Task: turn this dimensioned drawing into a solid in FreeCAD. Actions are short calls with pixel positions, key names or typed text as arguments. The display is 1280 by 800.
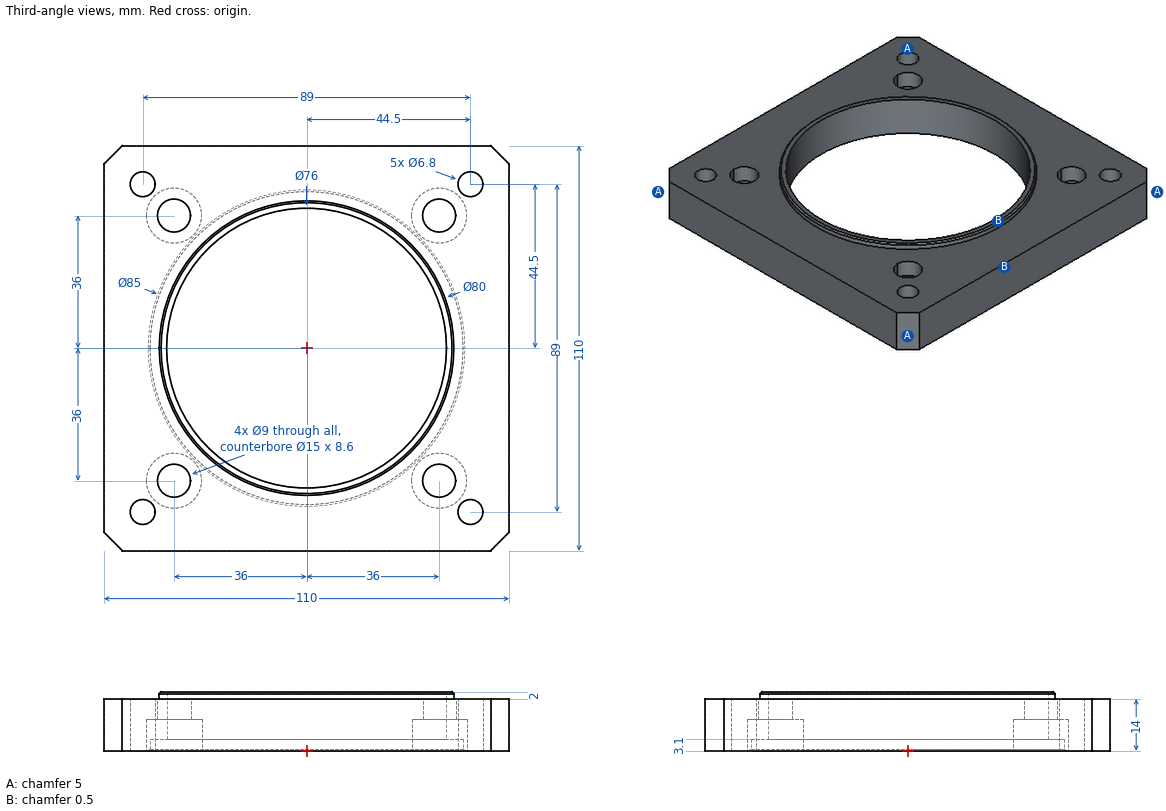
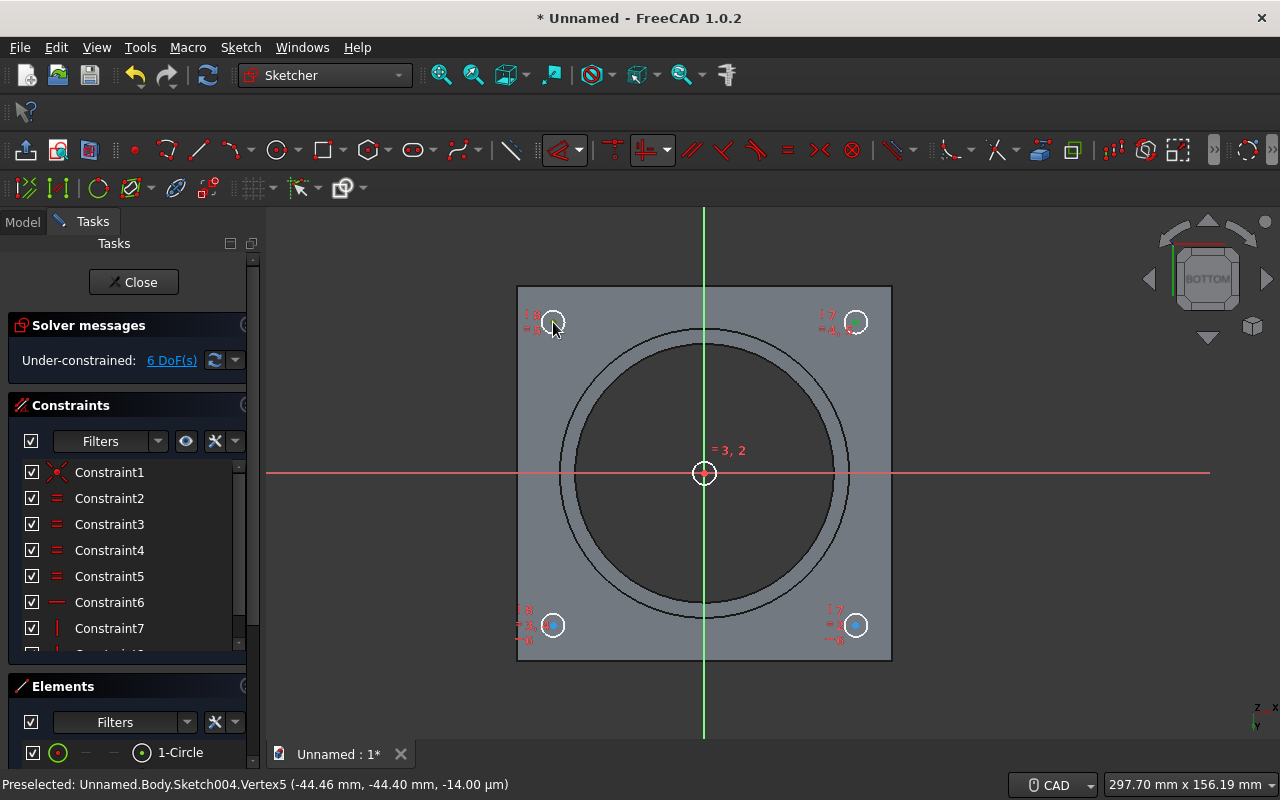
key(h)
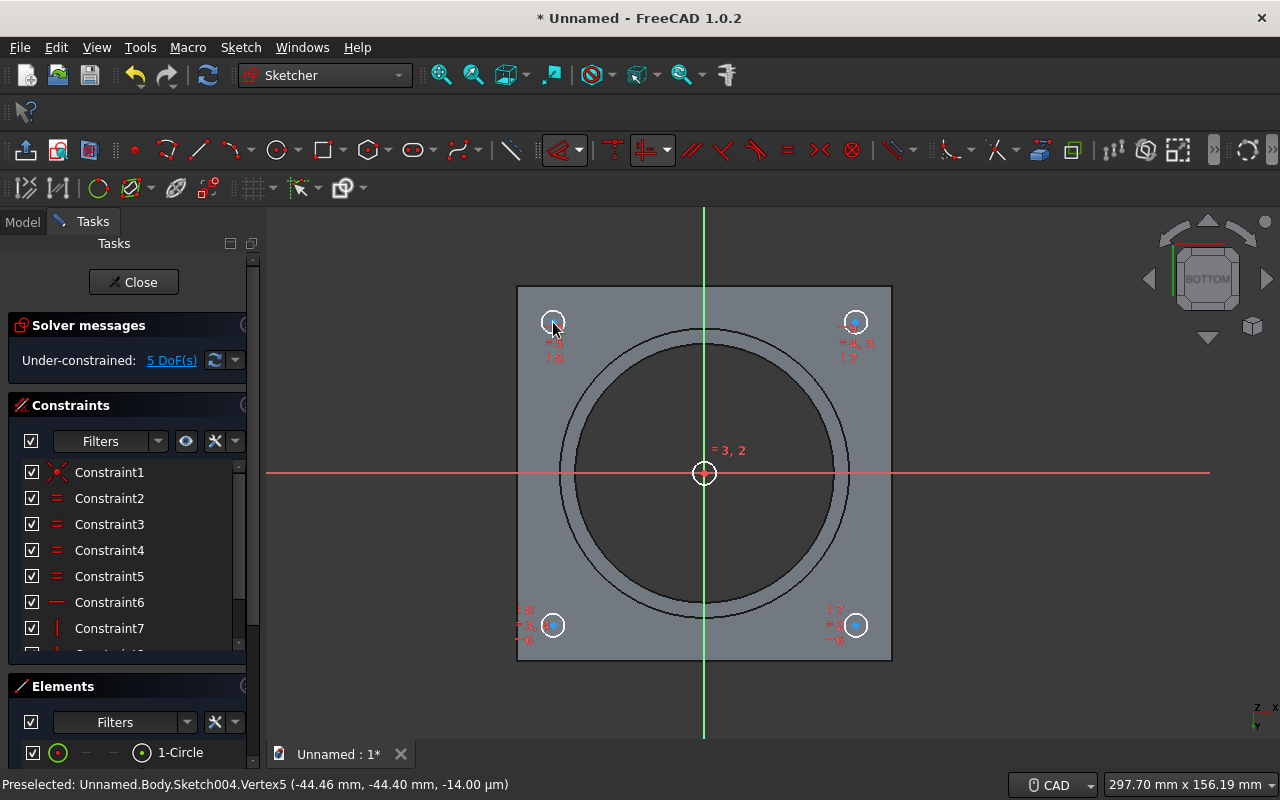
scroll(864, 617, up, 3)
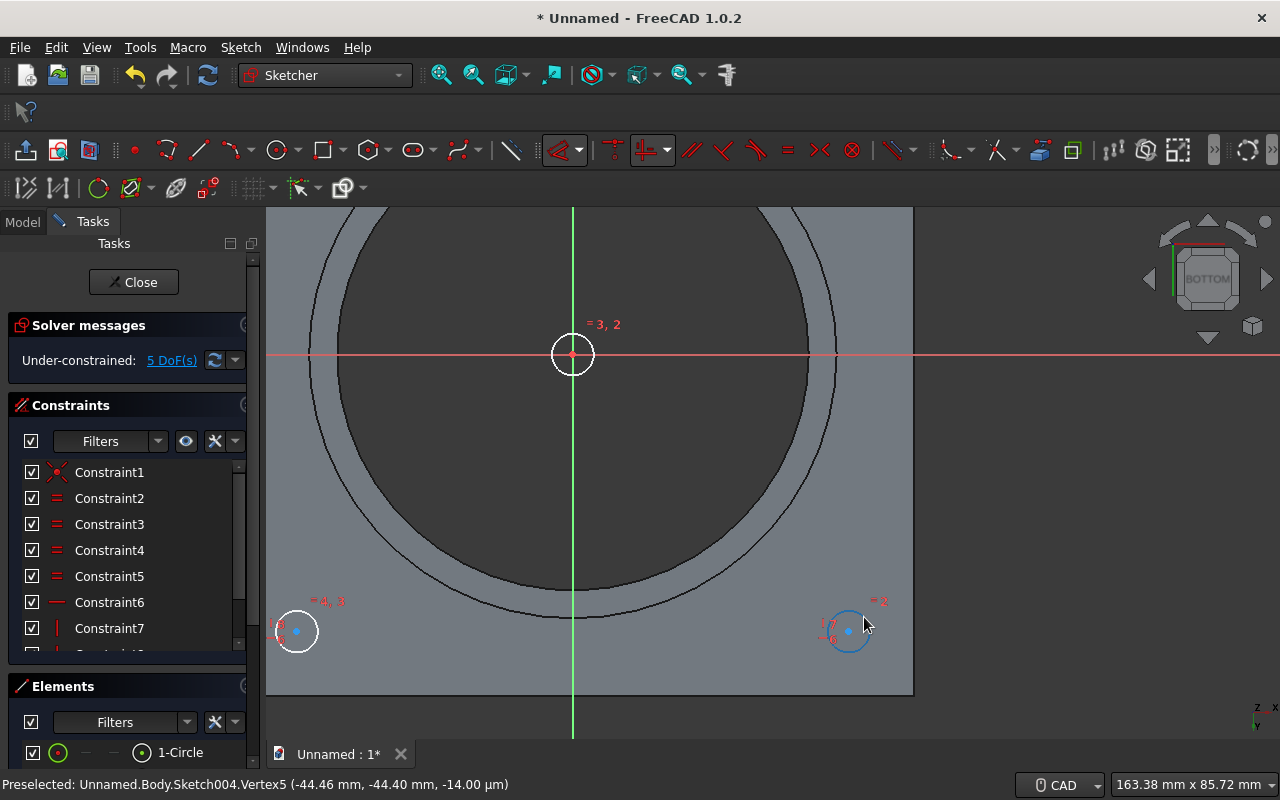
click(864, 617)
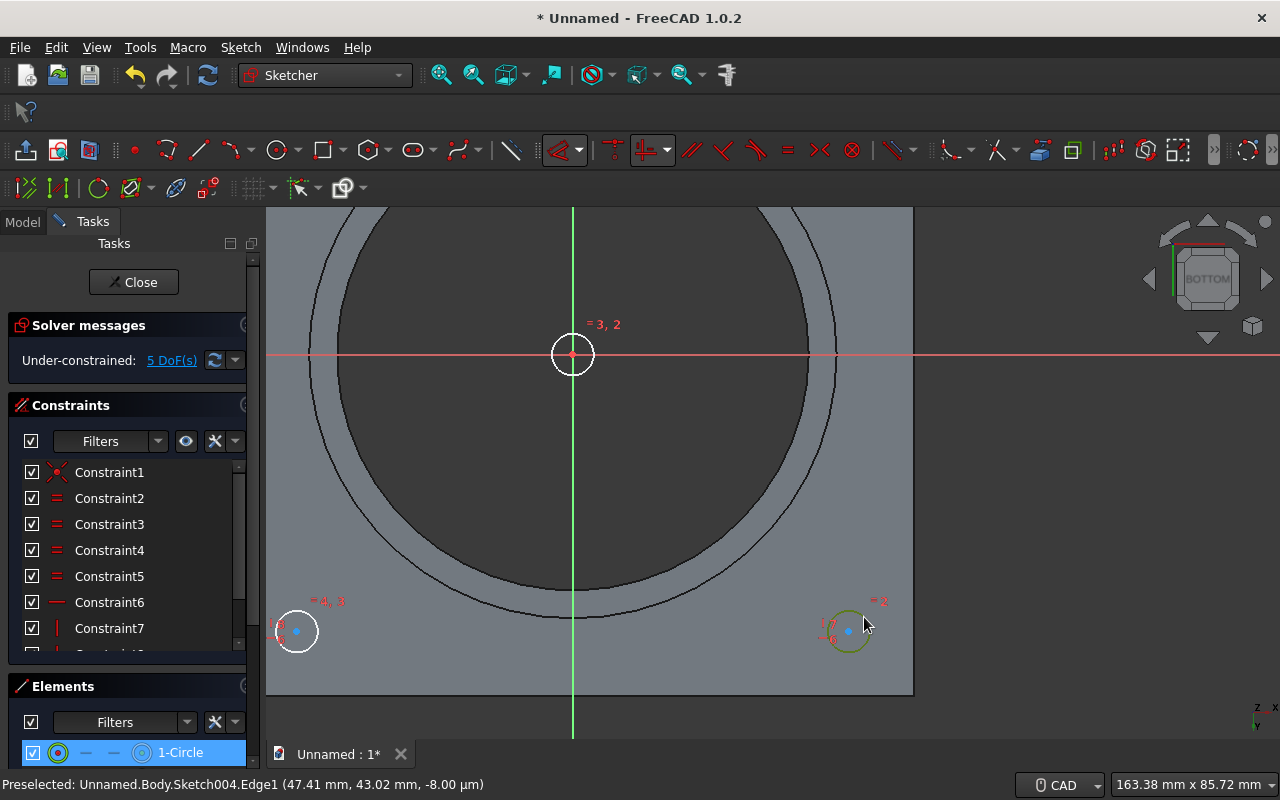
key(k)
key(o)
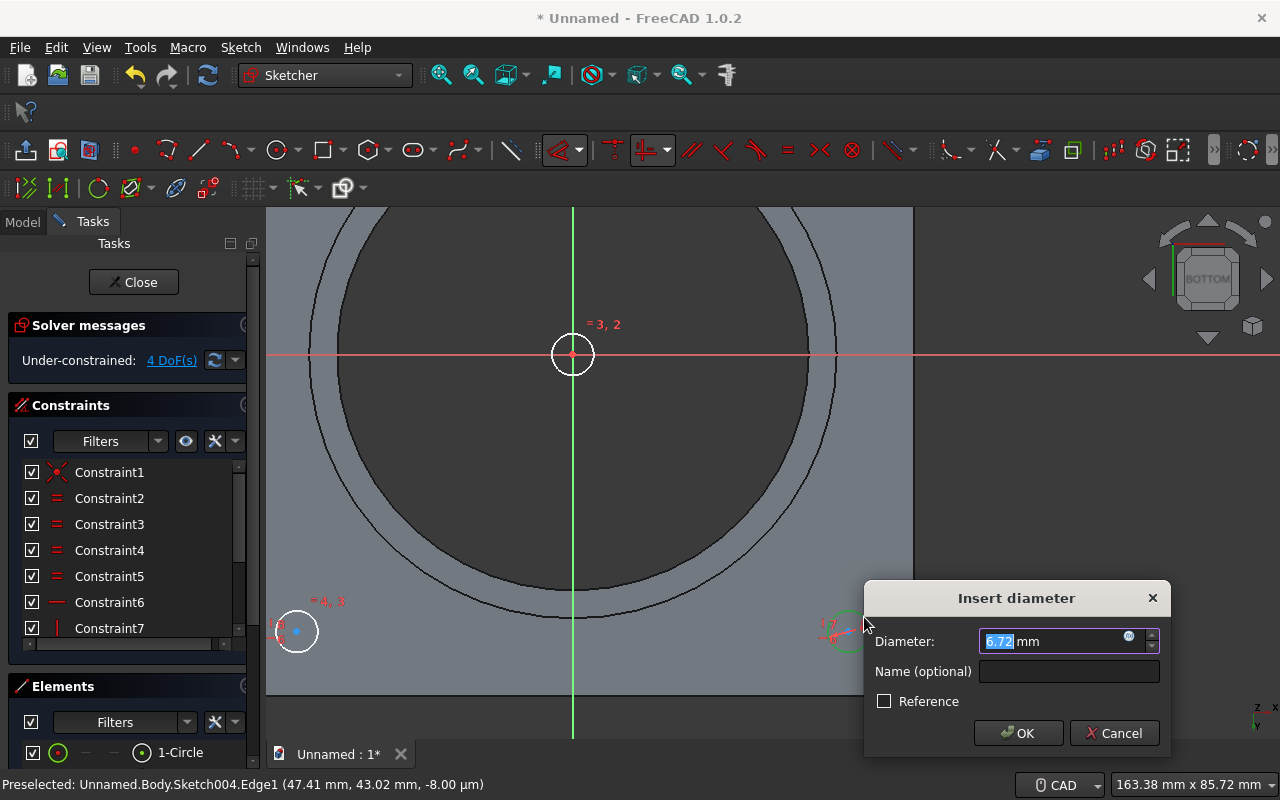
text(6.8)
key(Return)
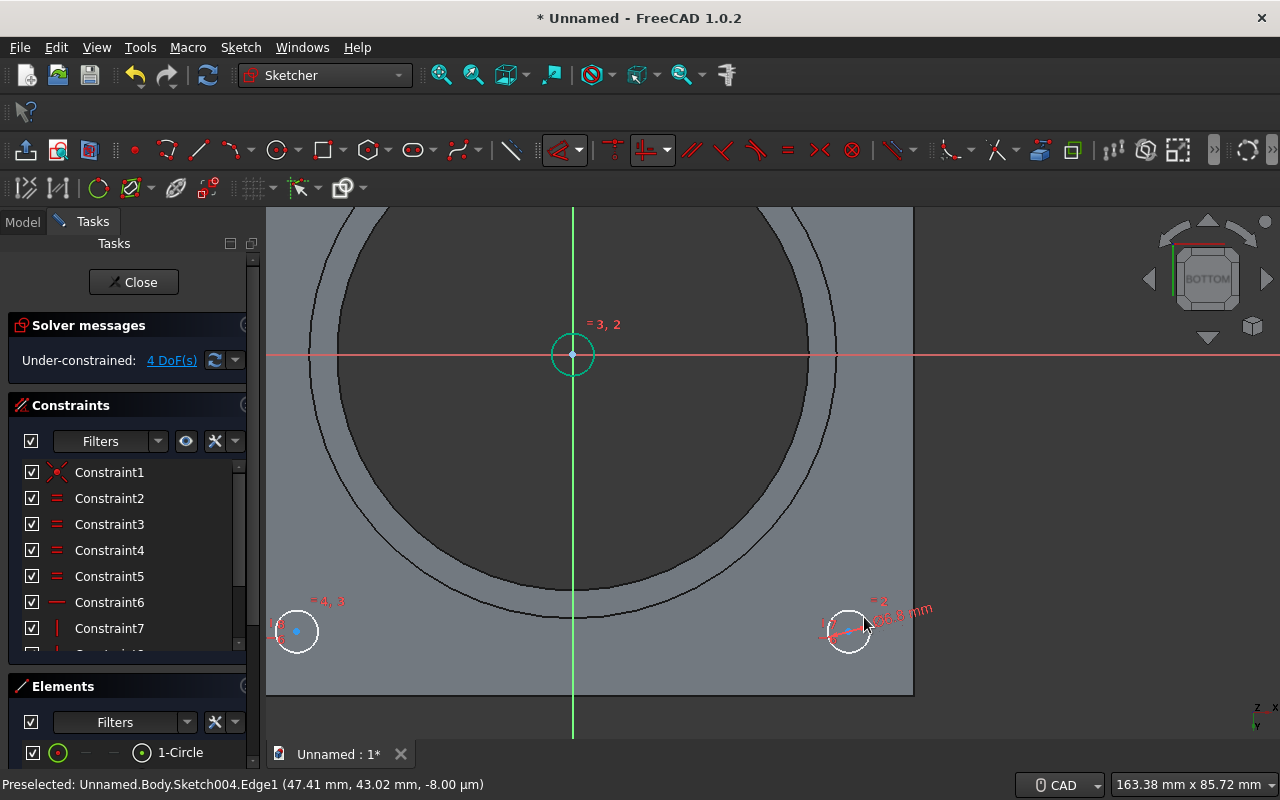
click(849, 632)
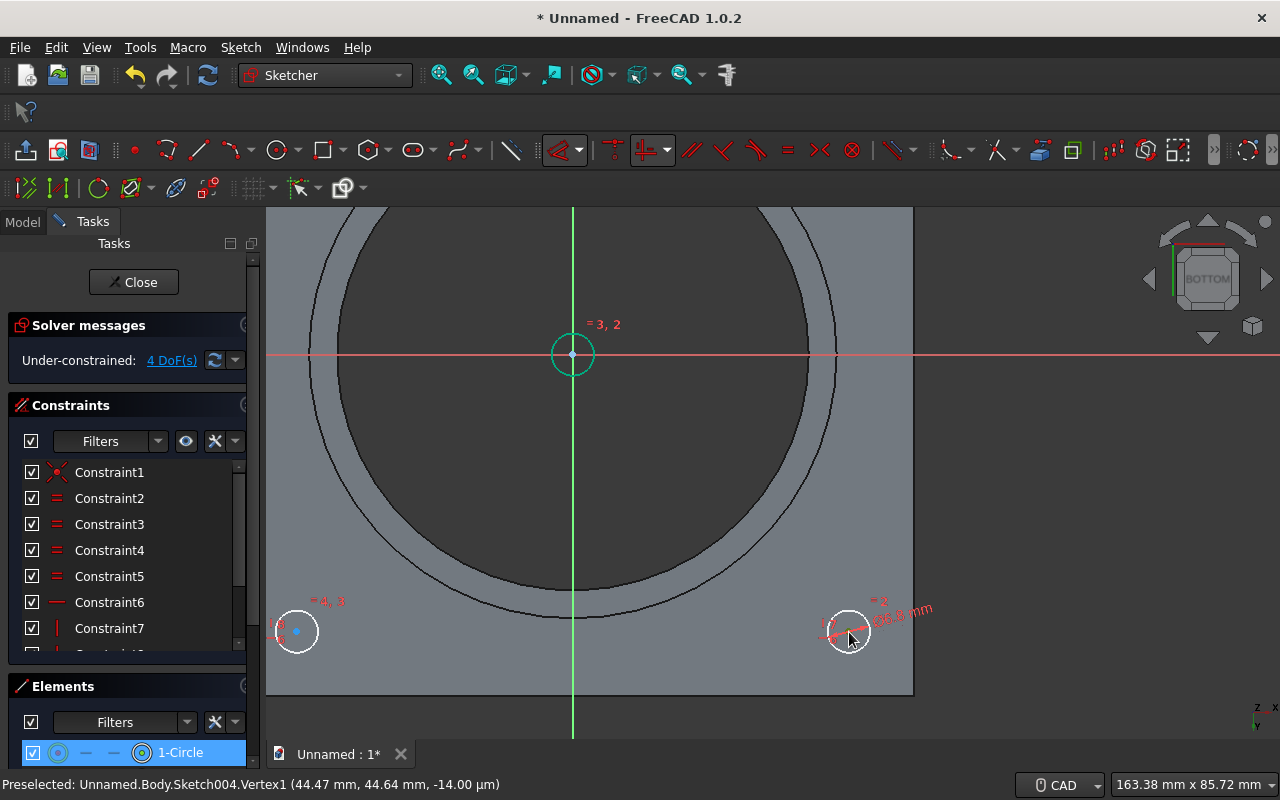
click(297, 632)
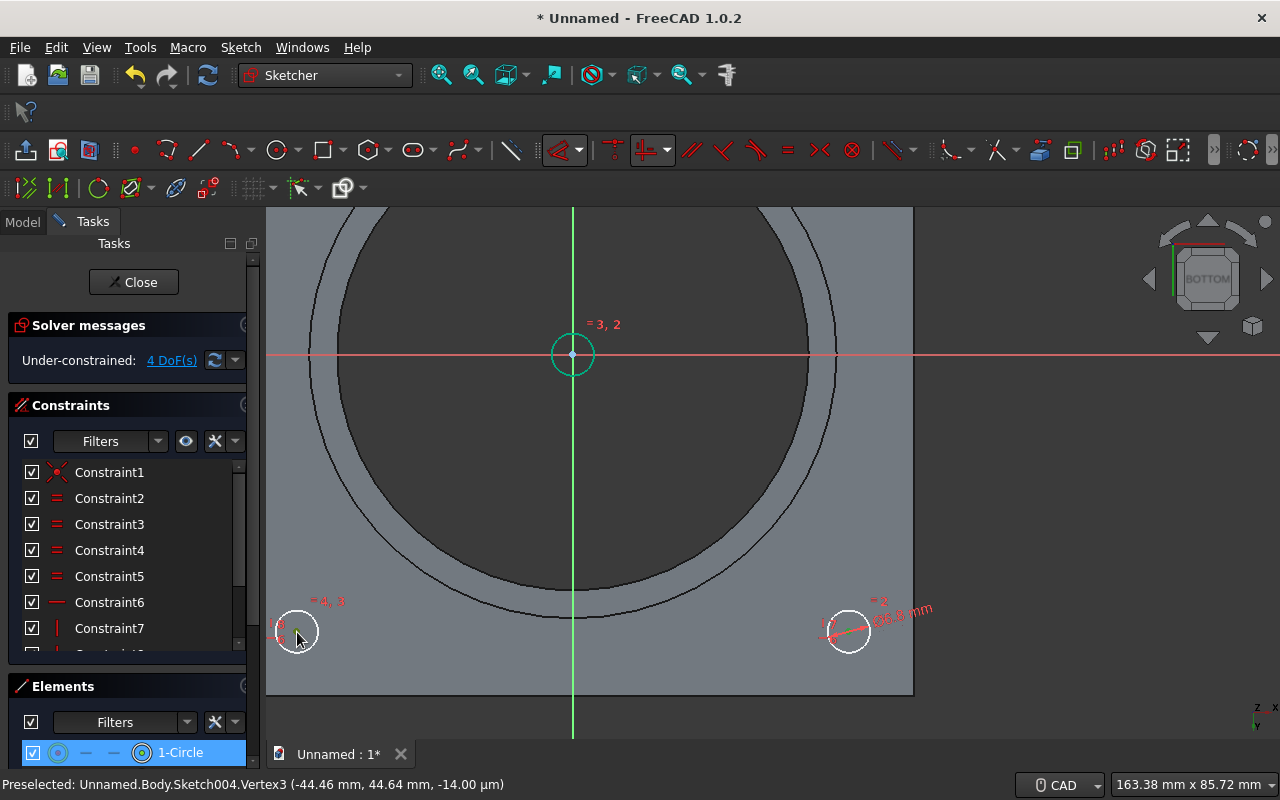
click(582, 150)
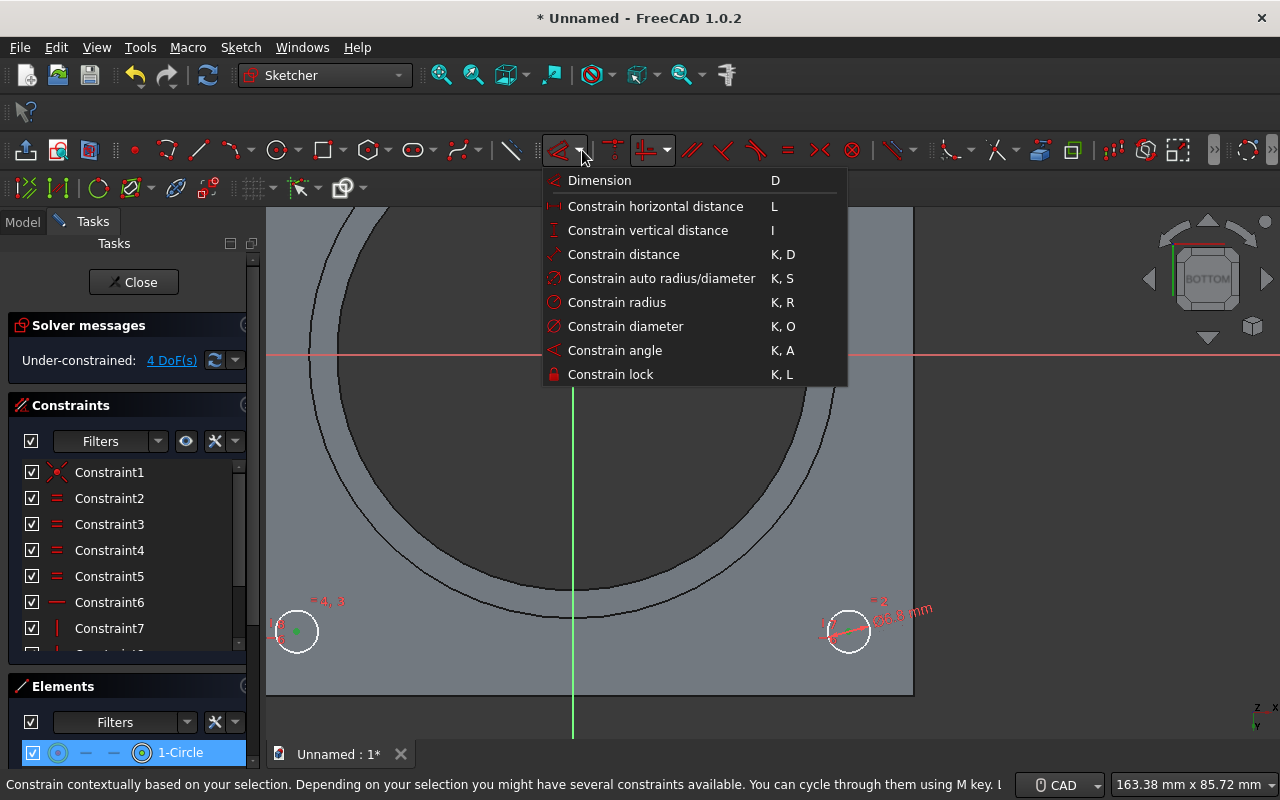
click(695, 206)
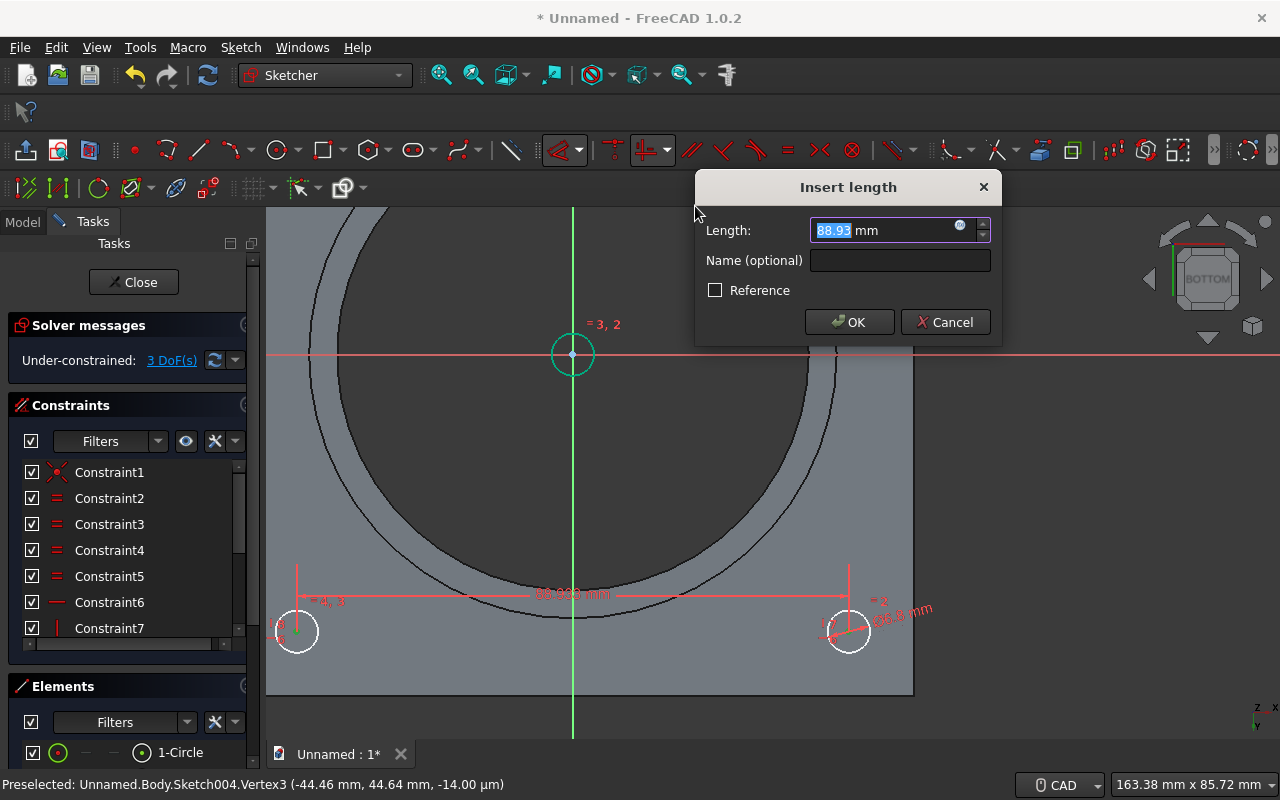
text(89)
key(Return)